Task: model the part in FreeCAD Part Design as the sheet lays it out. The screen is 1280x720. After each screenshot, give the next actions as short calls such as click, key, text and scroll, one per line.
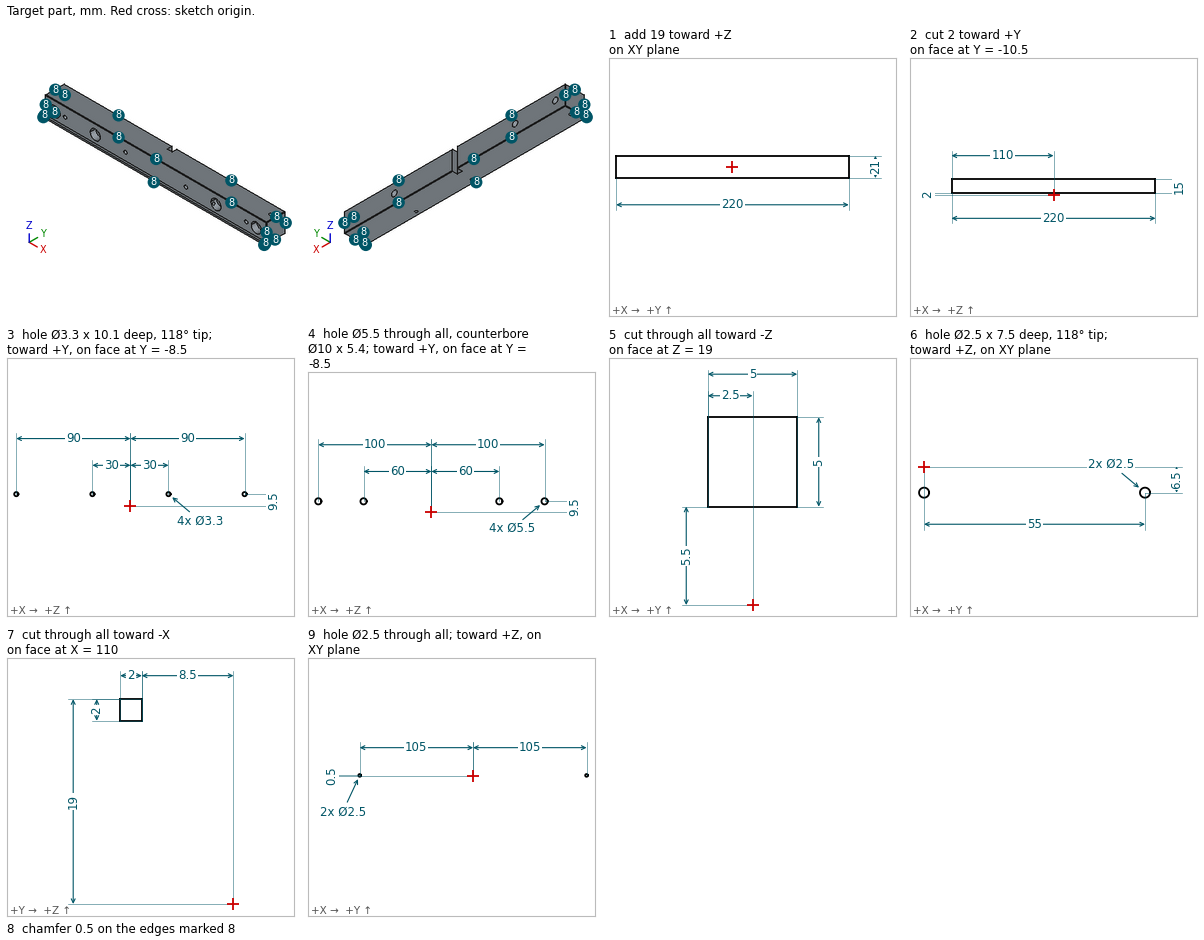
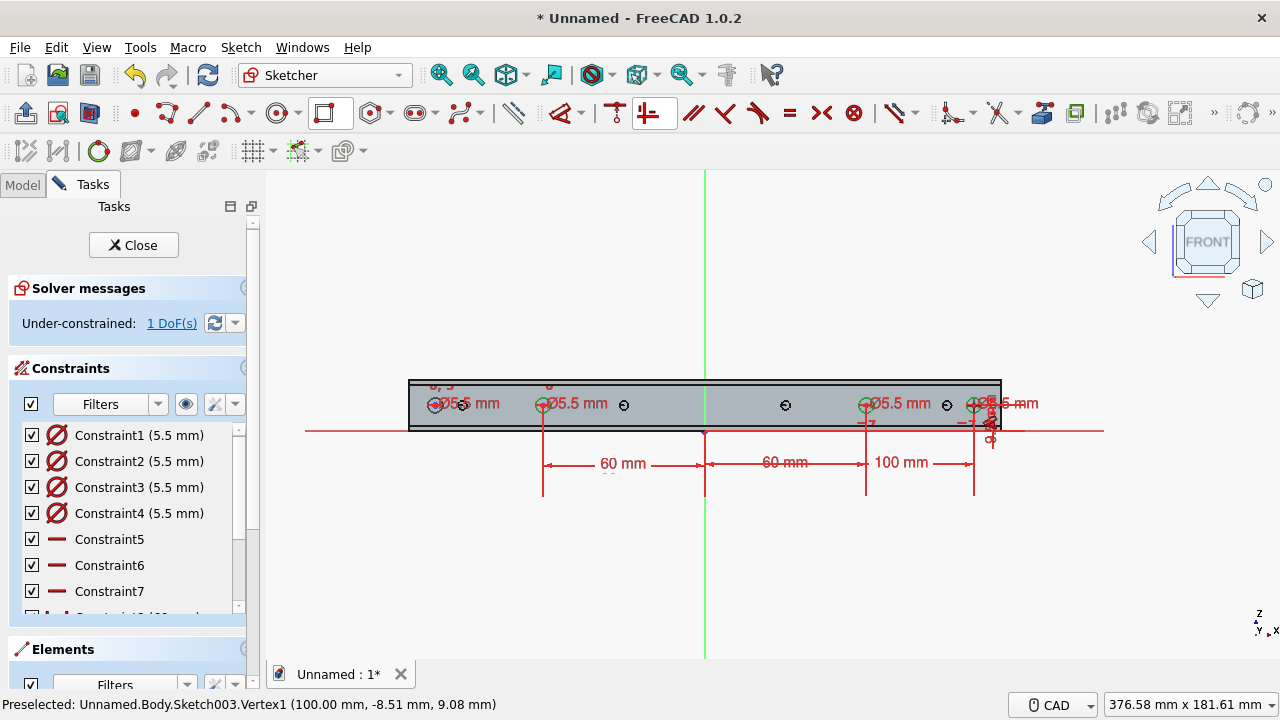
click(435, 405)
click(508, 465)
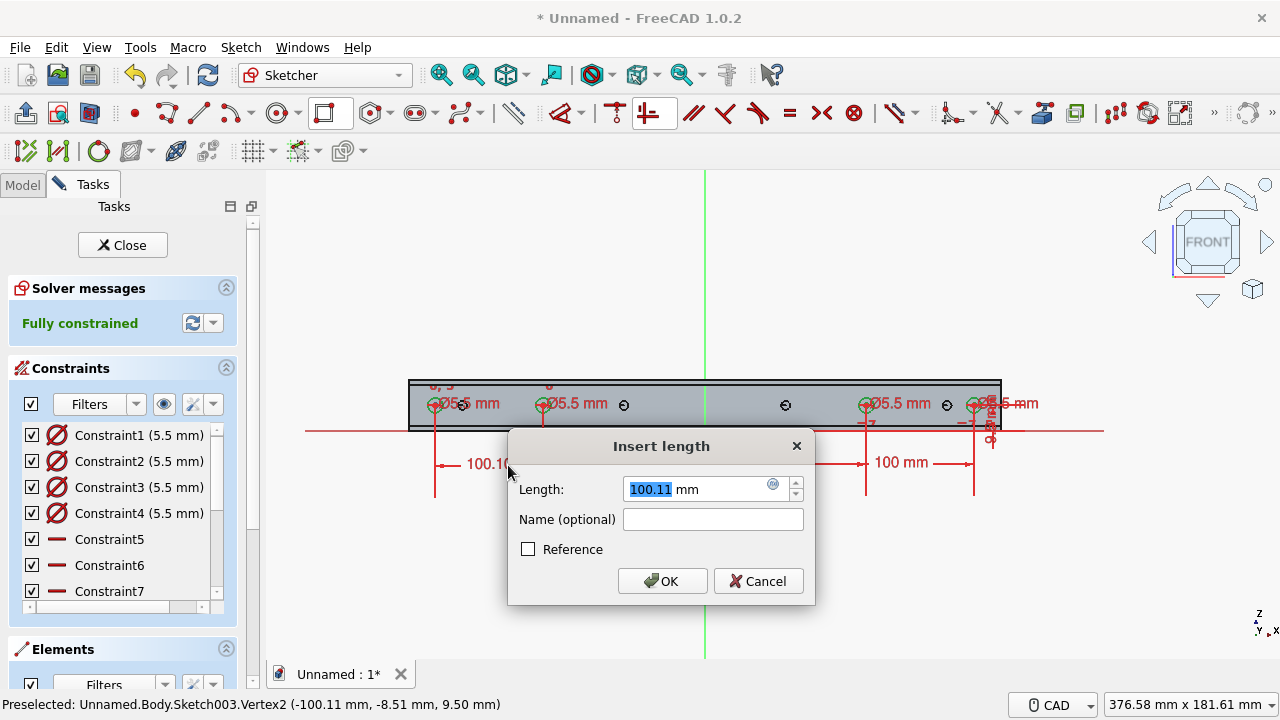
text(100)
key(Return)
key(Escape)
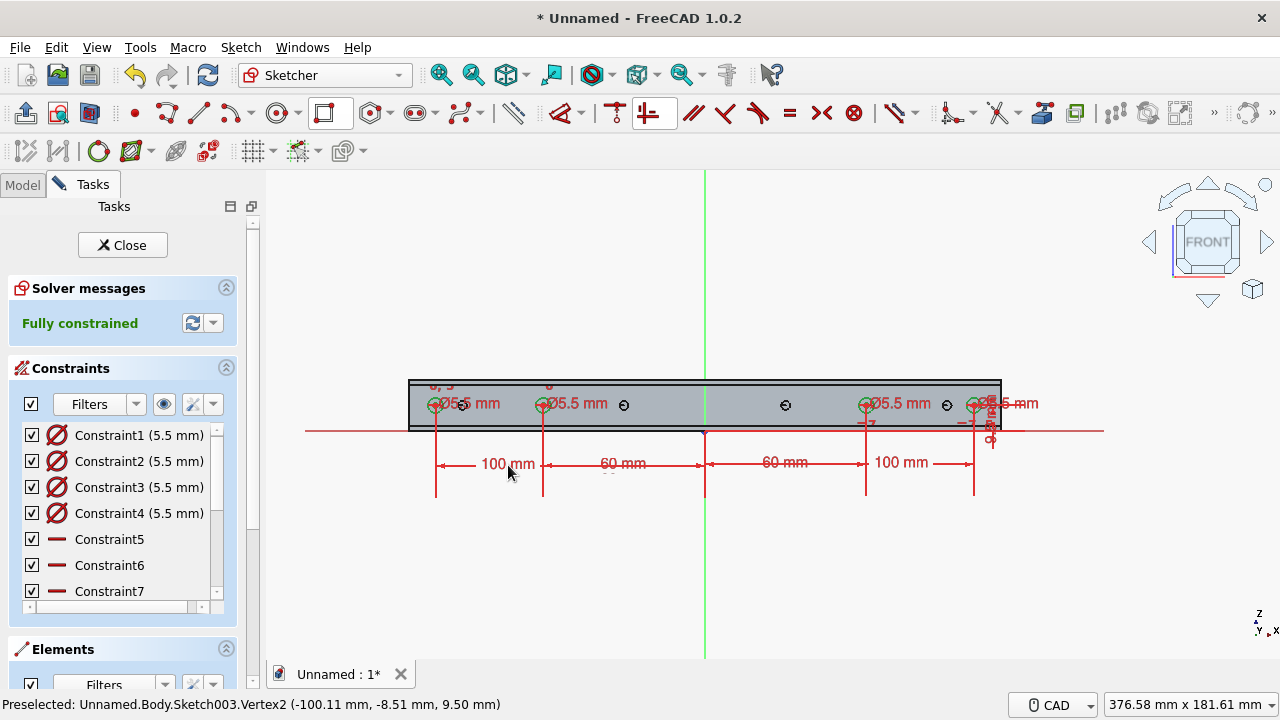
click(123, 245)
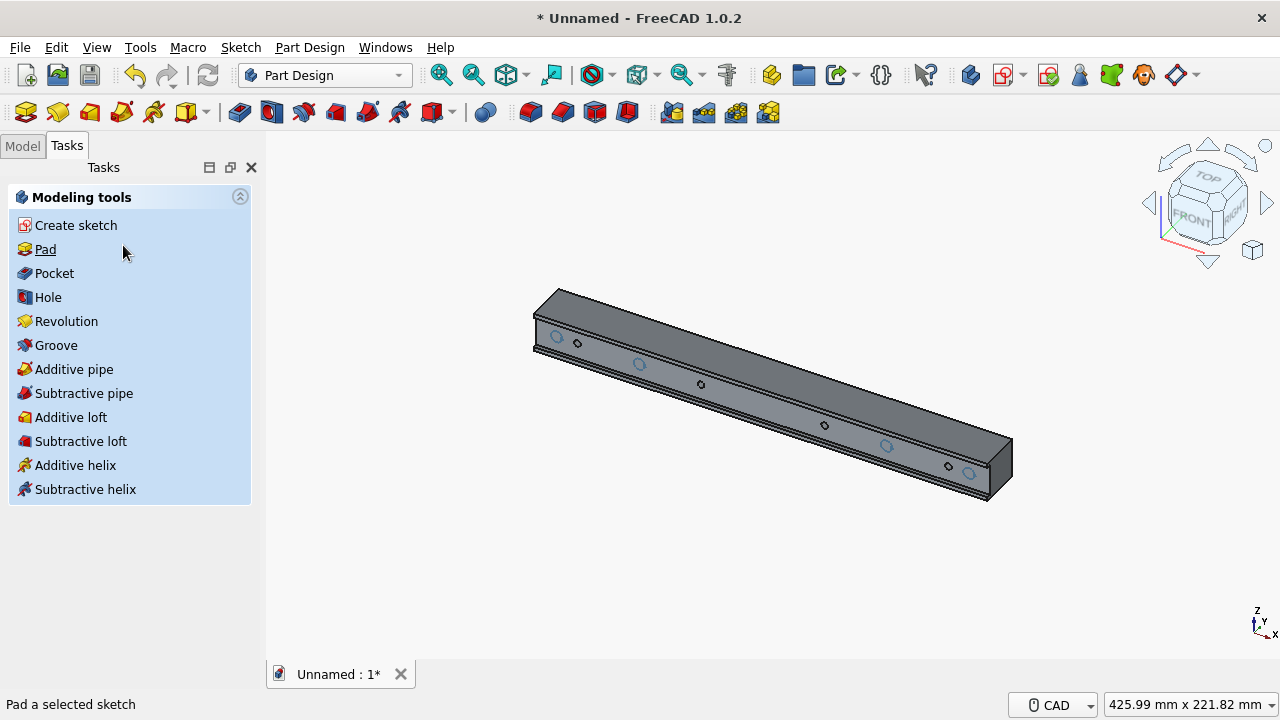
click(272, 112)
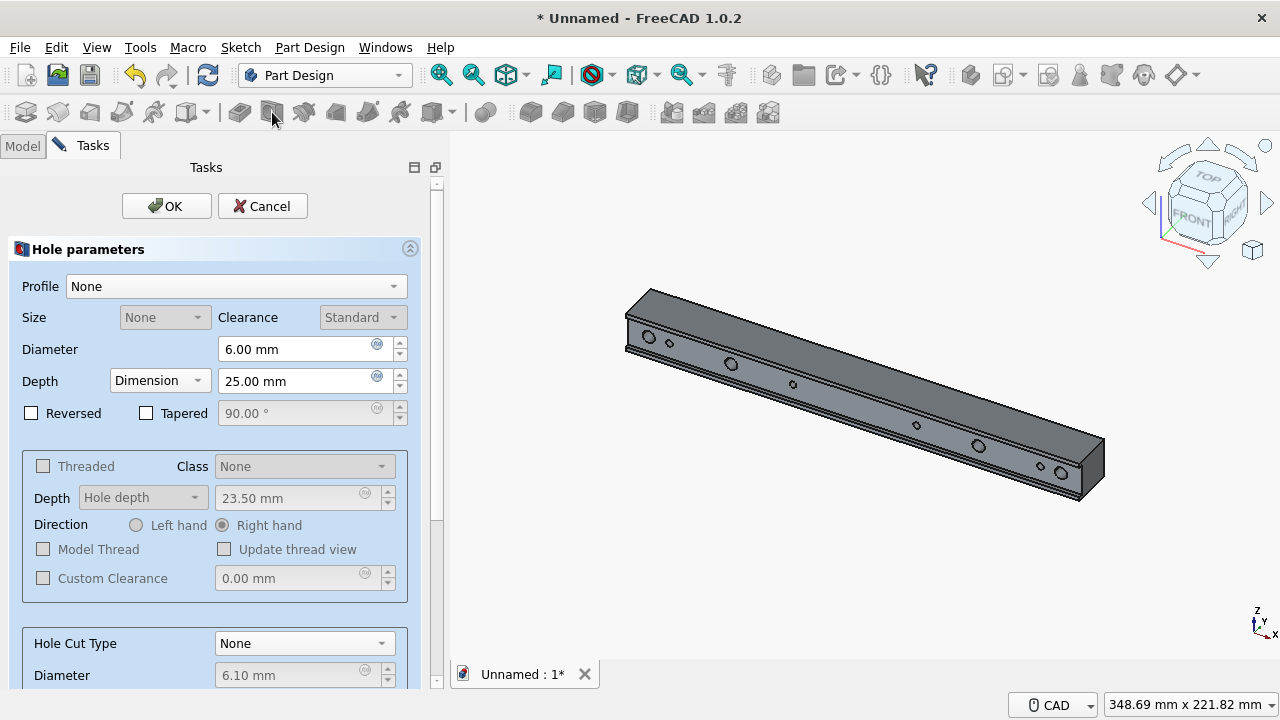
triple_click(305, 349)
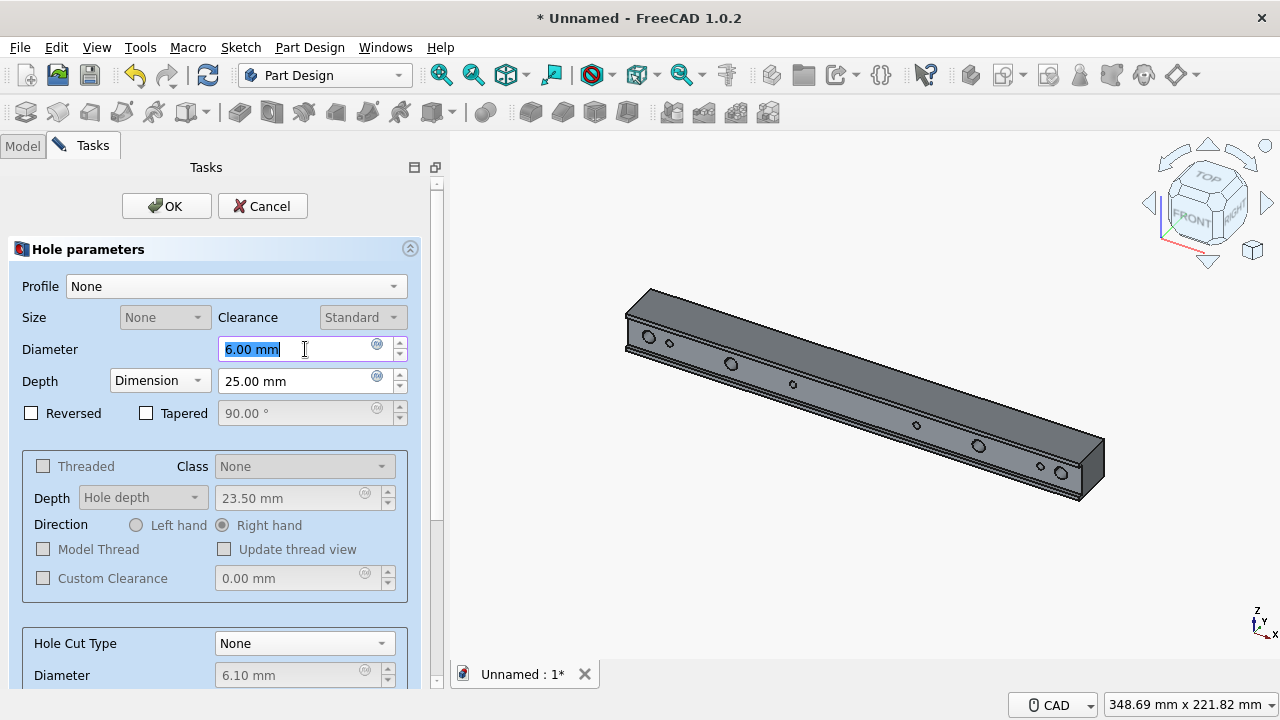
text(5.5)
key(Tab)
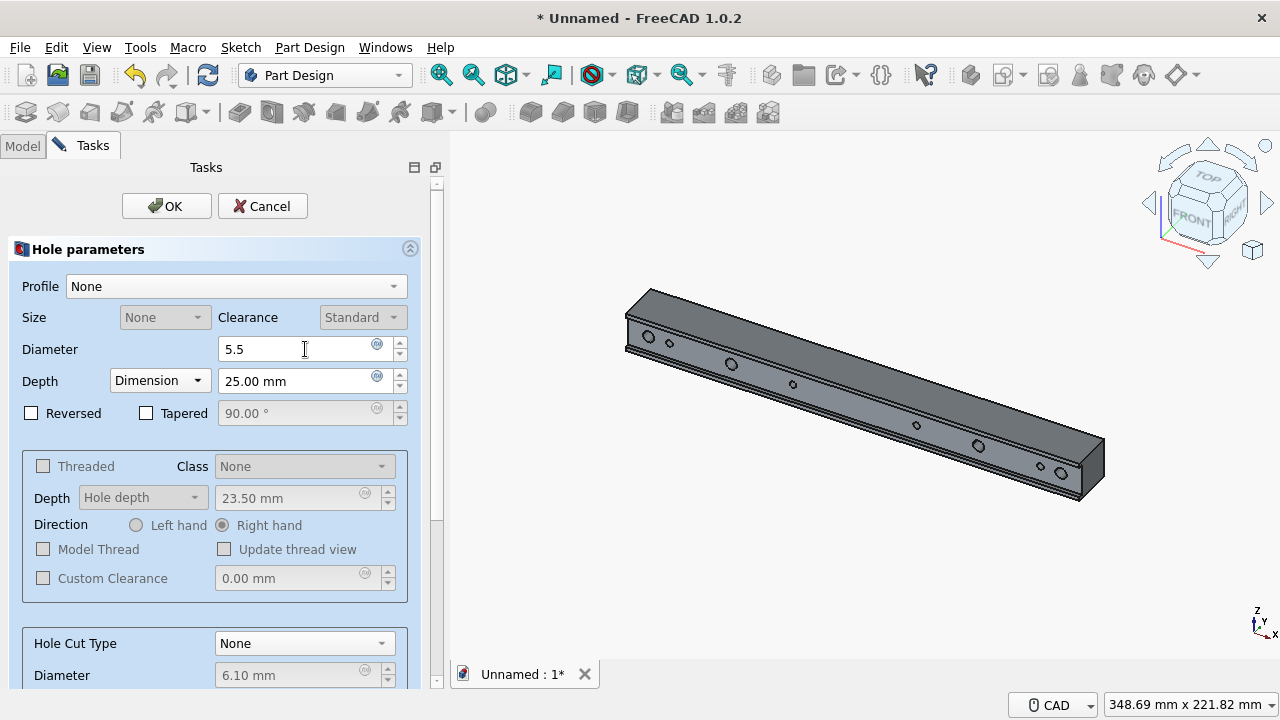
click(161, 380)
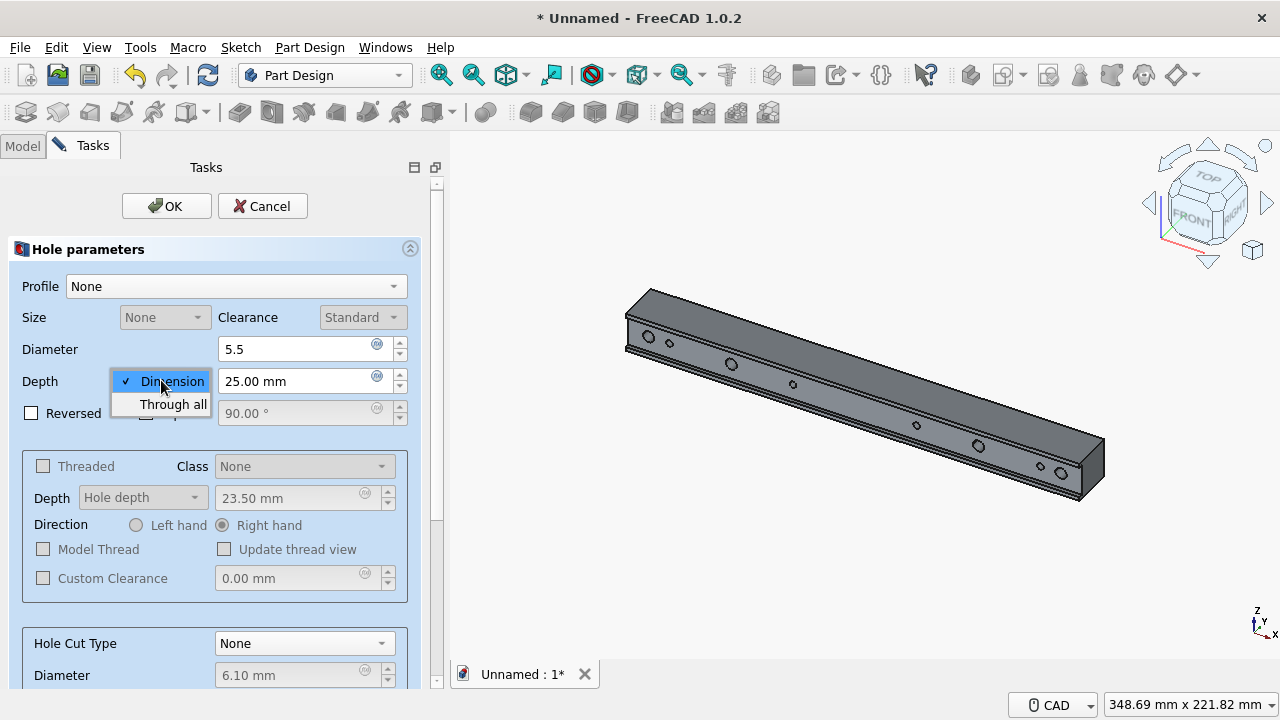
click(160, 404)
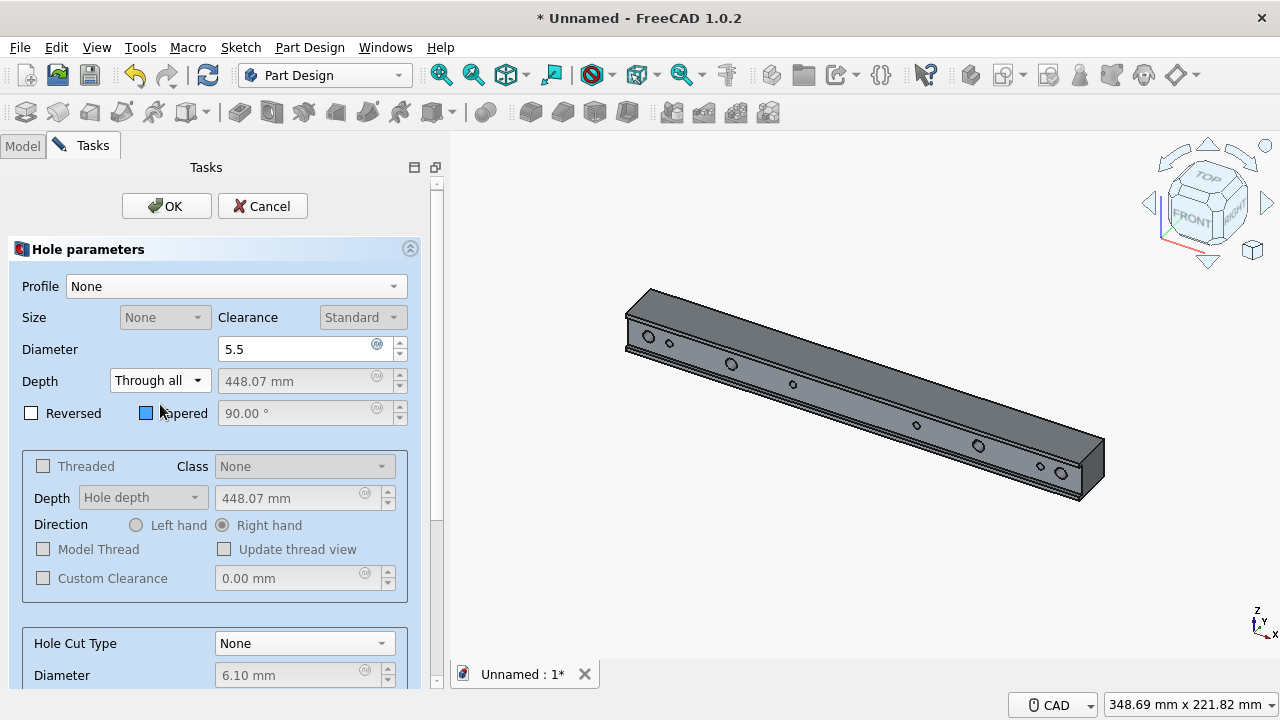
click(306, 644)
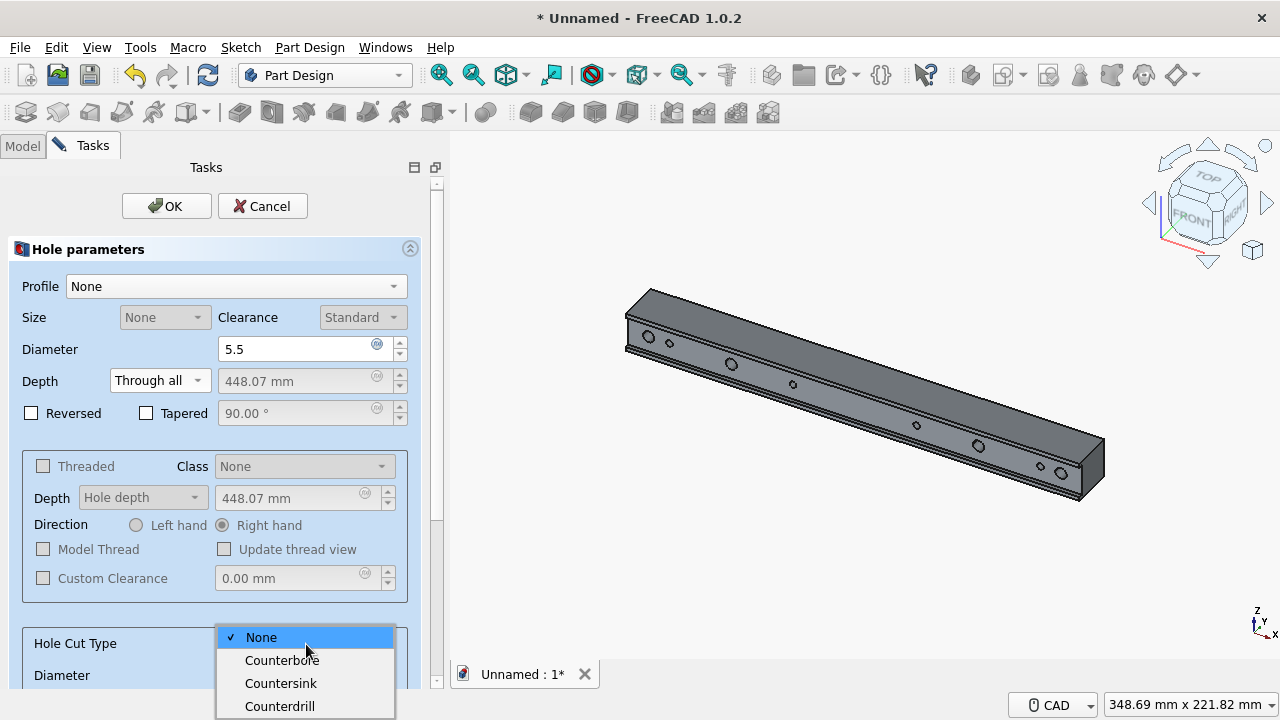
click(304, 660)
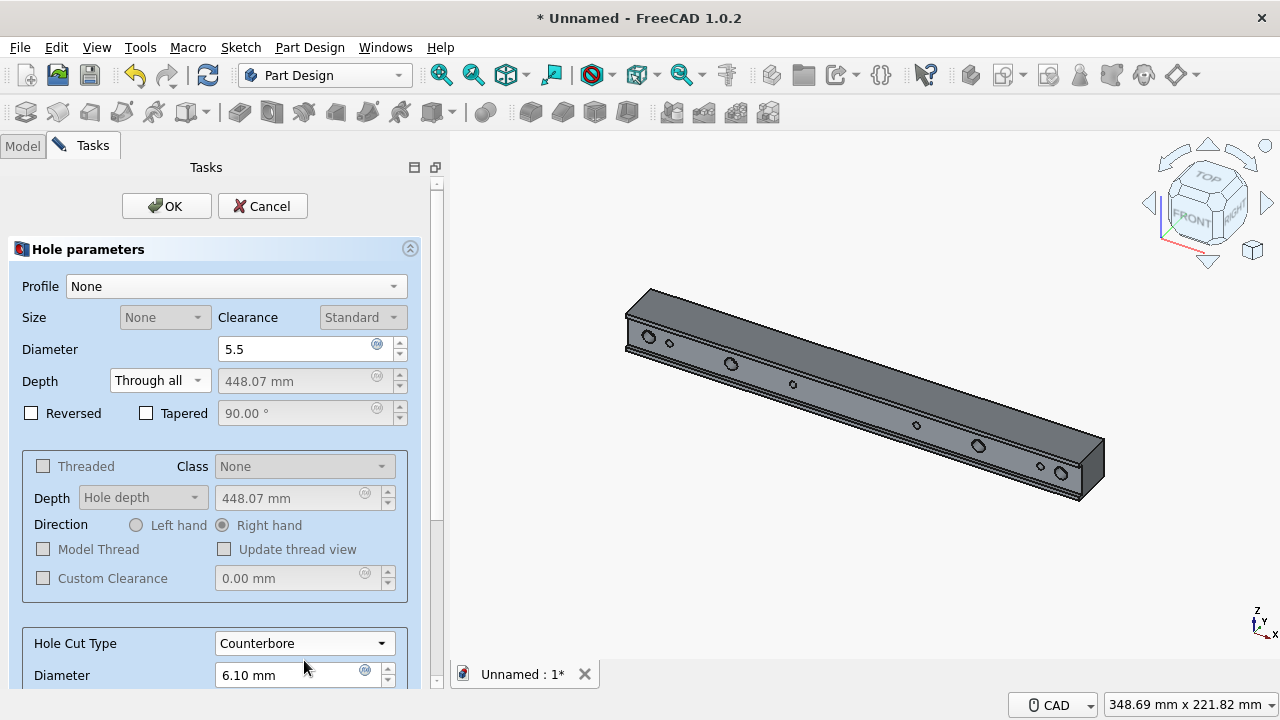
triple_click(298, 675)